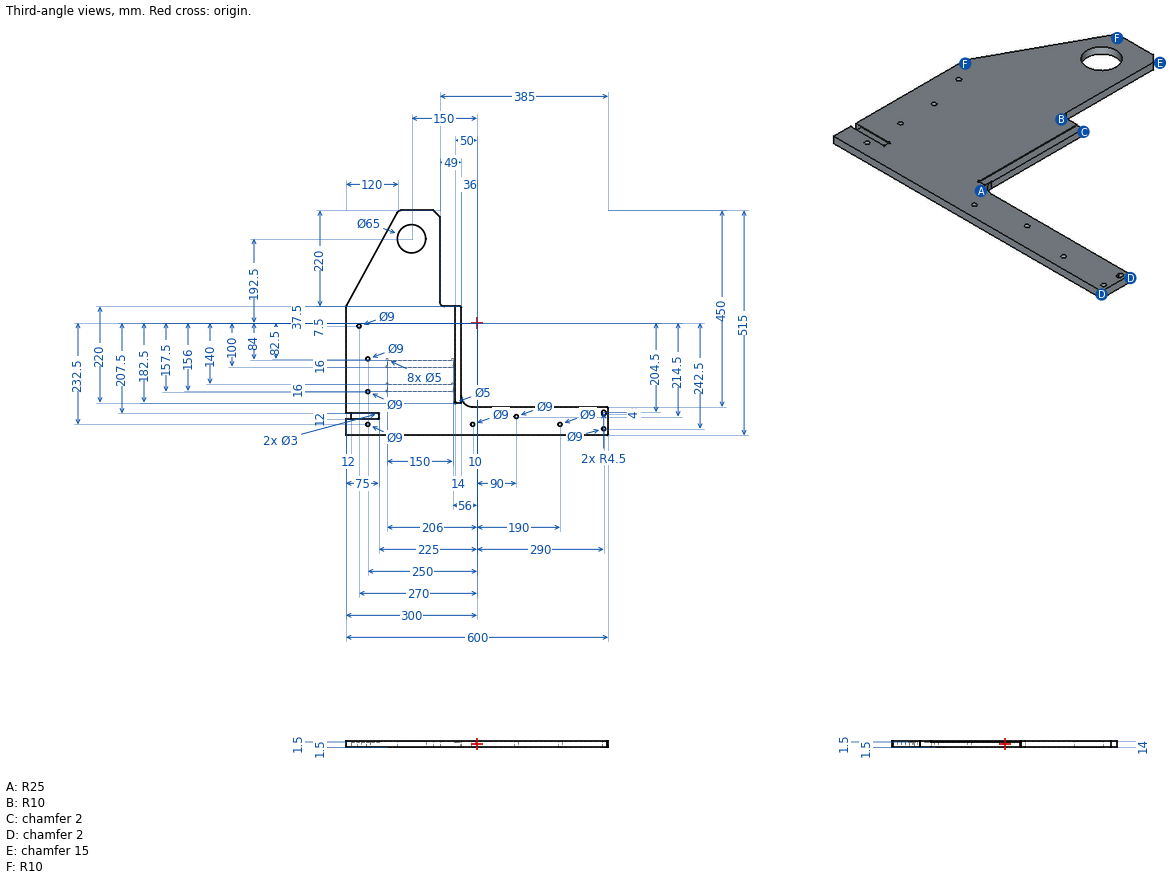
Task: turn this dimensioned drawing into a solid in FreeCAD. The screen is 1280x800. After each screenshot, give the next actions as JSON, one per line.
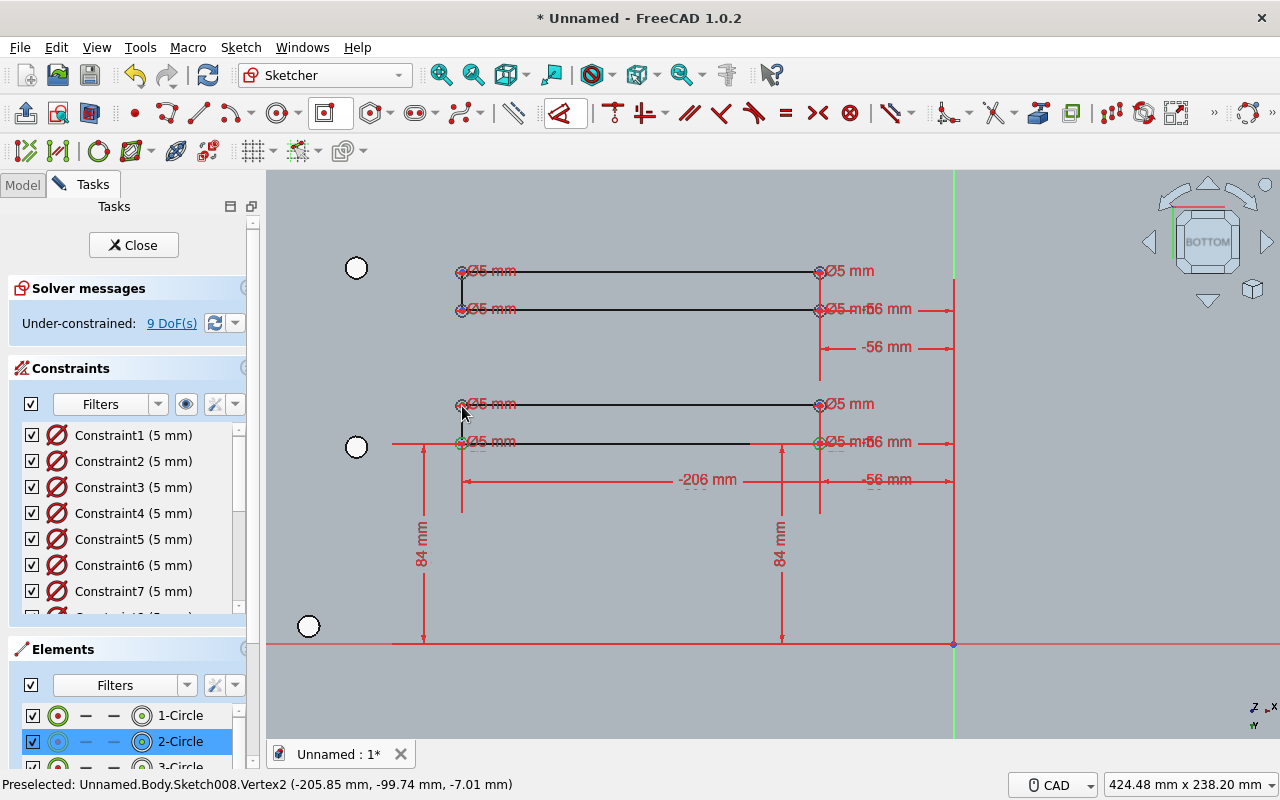
{"action": "left_click", "coordinate": [582, 114]}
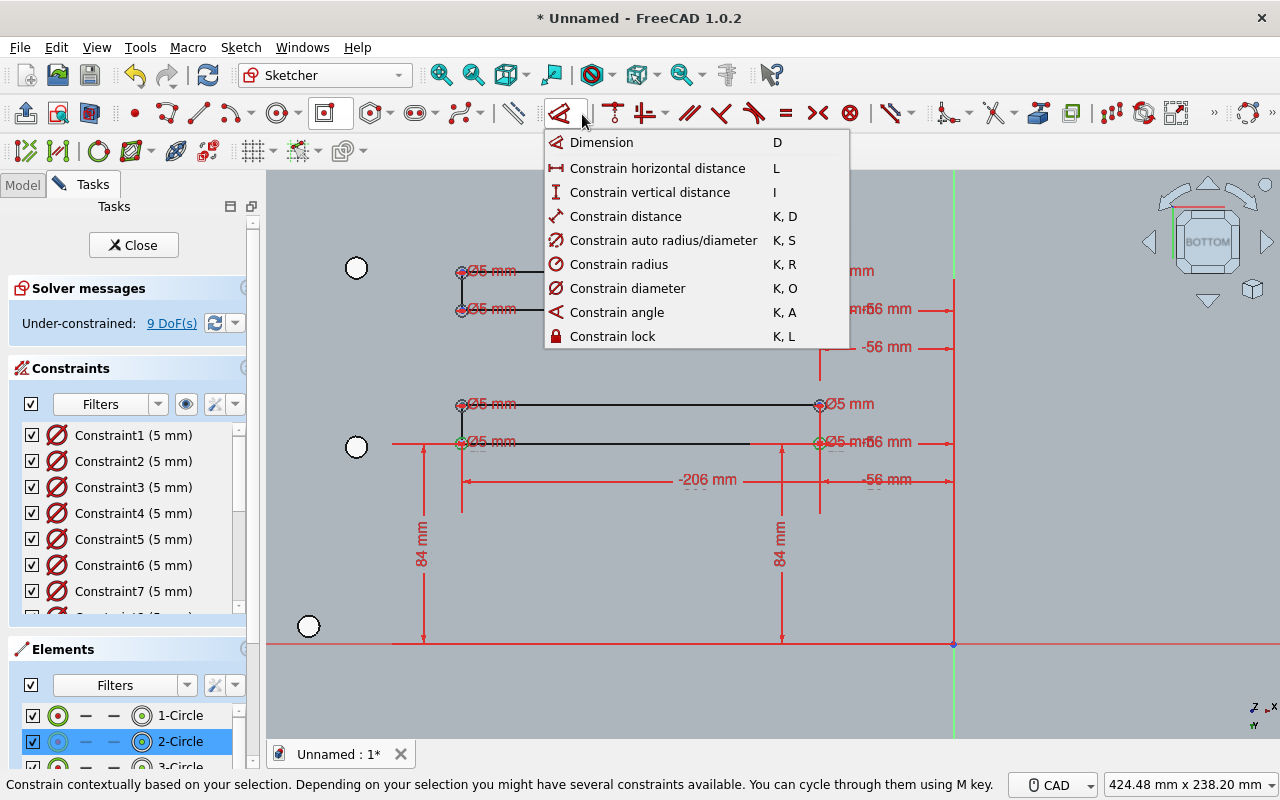
{"action": "left_click", "coordinate": [697, 168]}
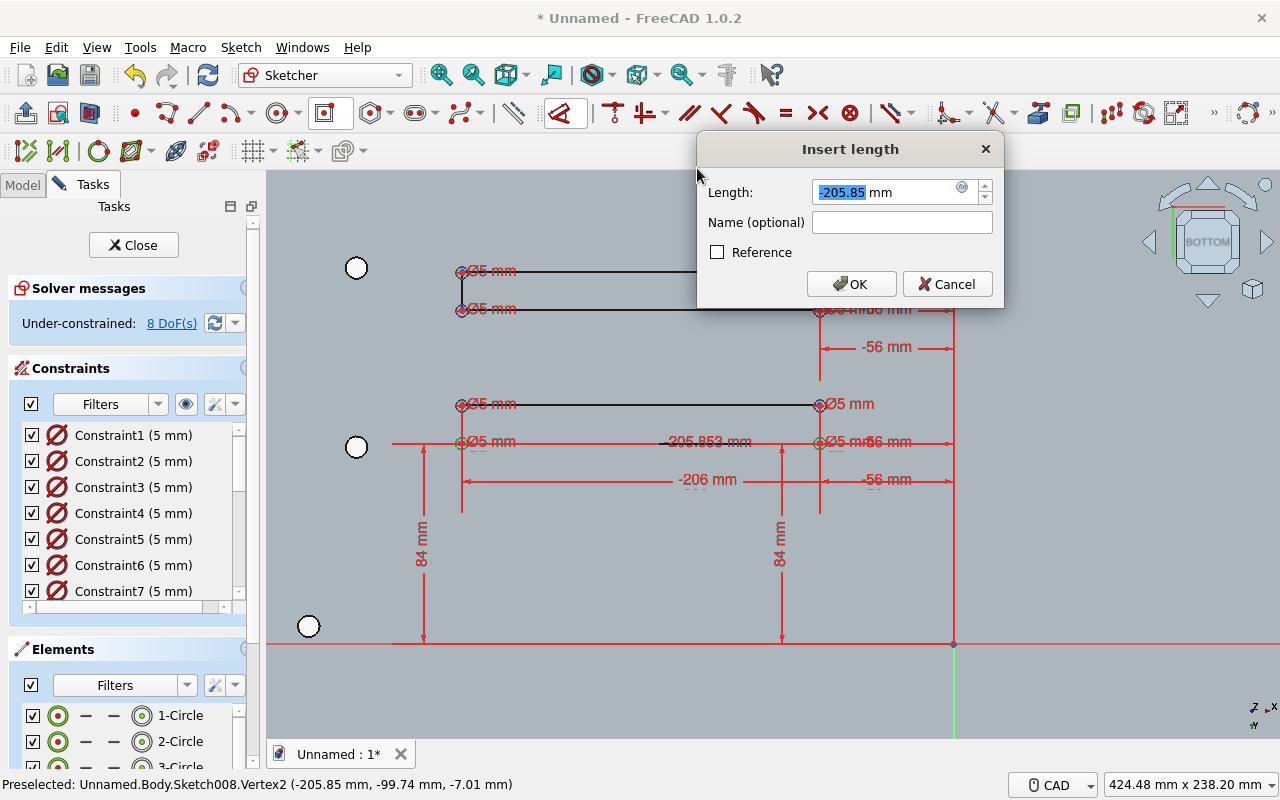
{"action": "type", "text": "-206"}
{"action": "key", "text": "Return"}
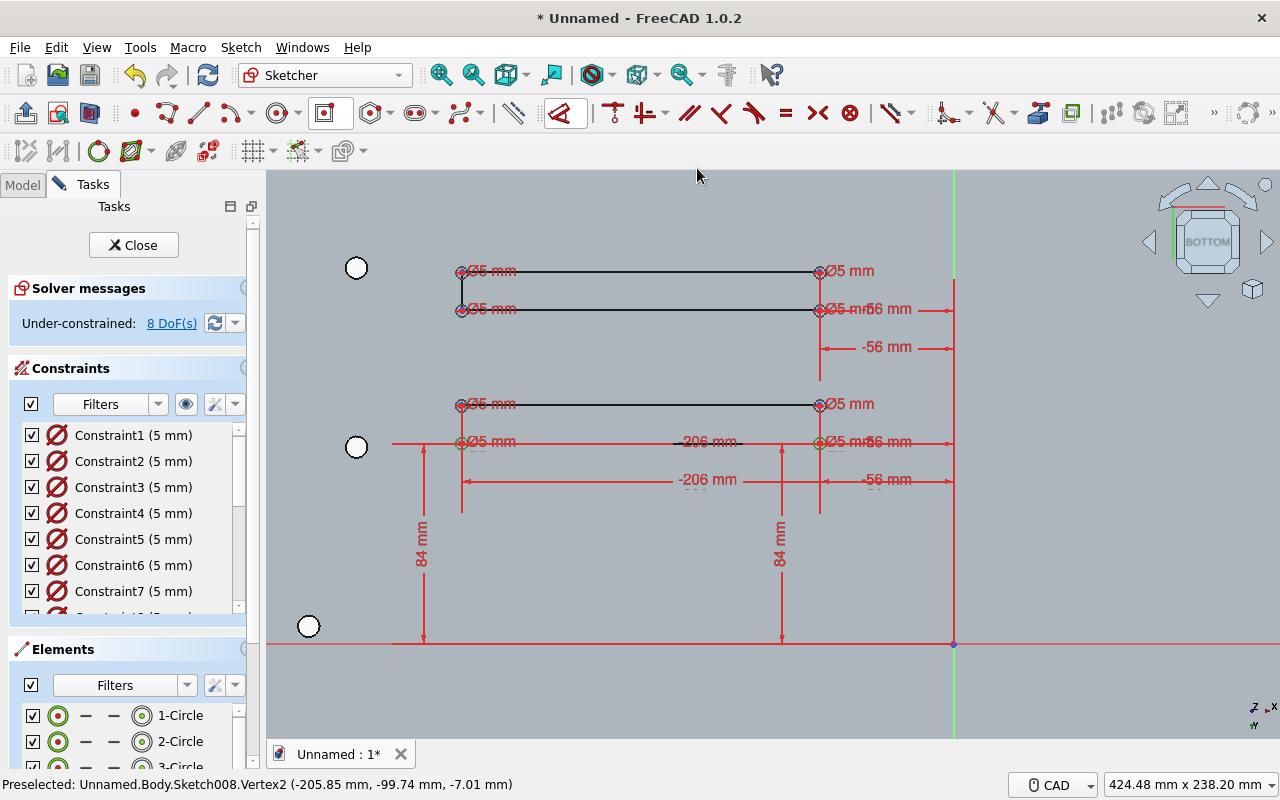
{"action": "left_click", "coordinate": [462, 406]}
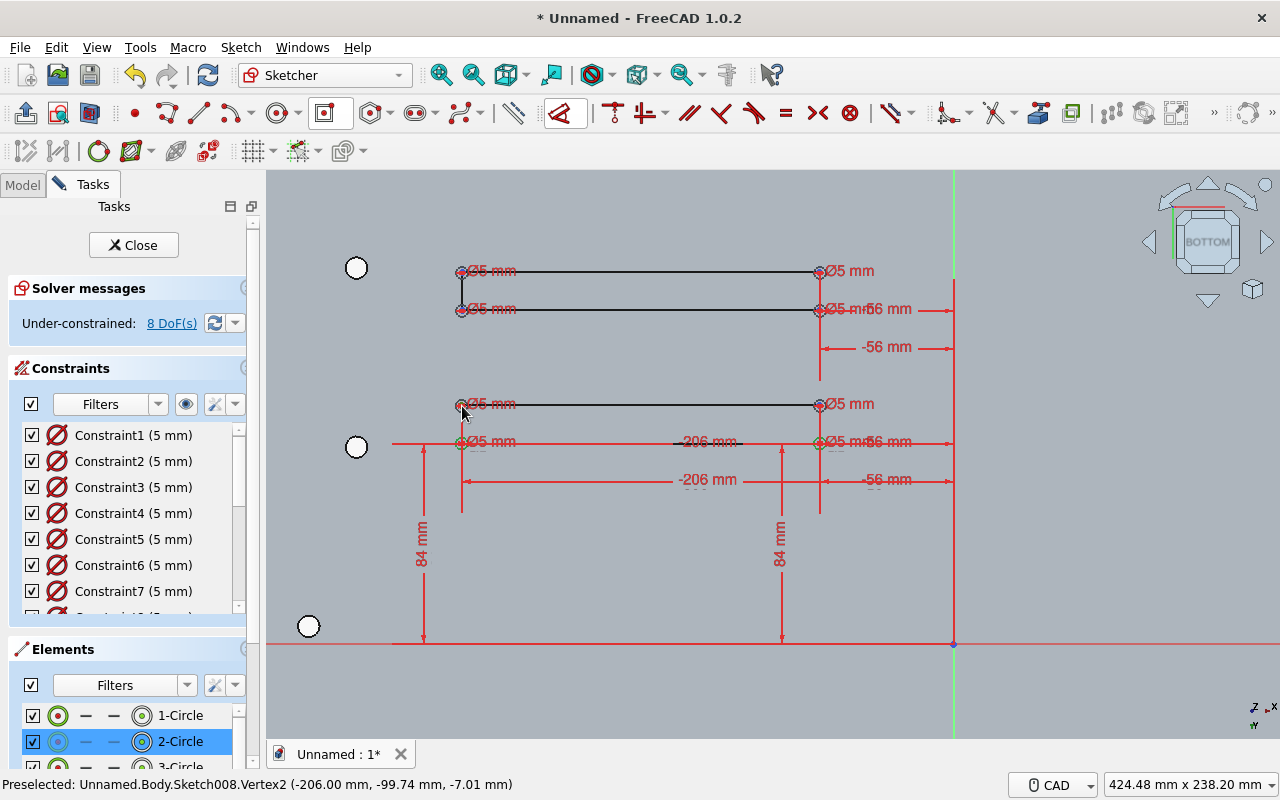
{"action": "left_click", "coordinate": [582, 114]}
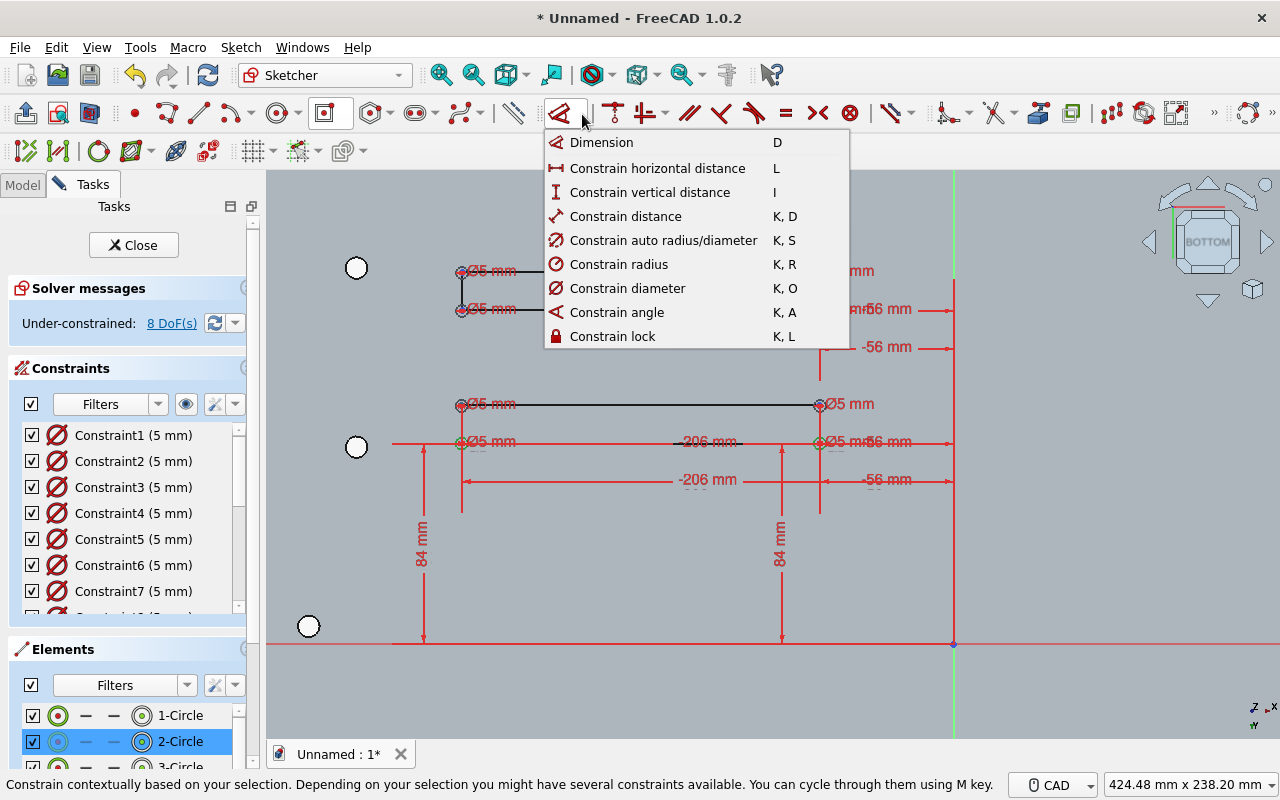
{"action": "left_click", "coordinate": [697, 192]}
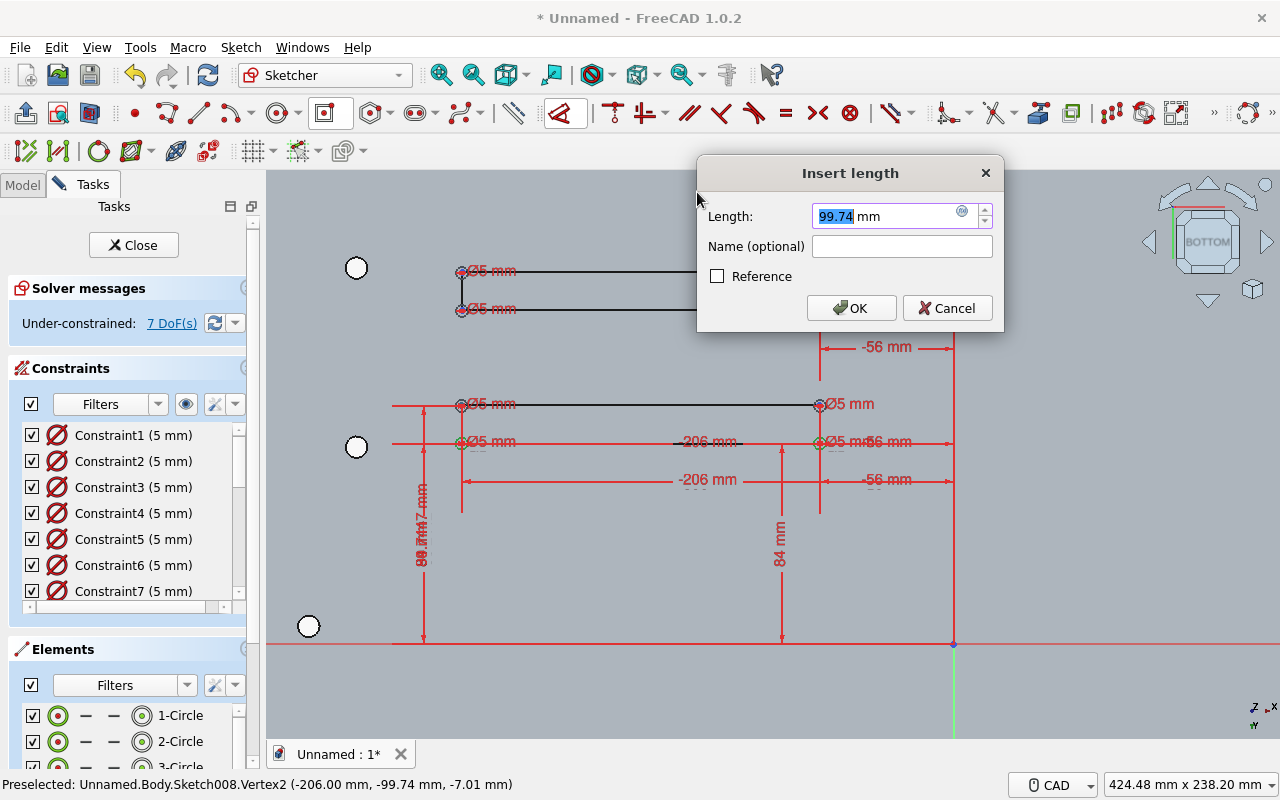
{"action": "type", "text": "100"}
{"action": "key", "text": "Return"}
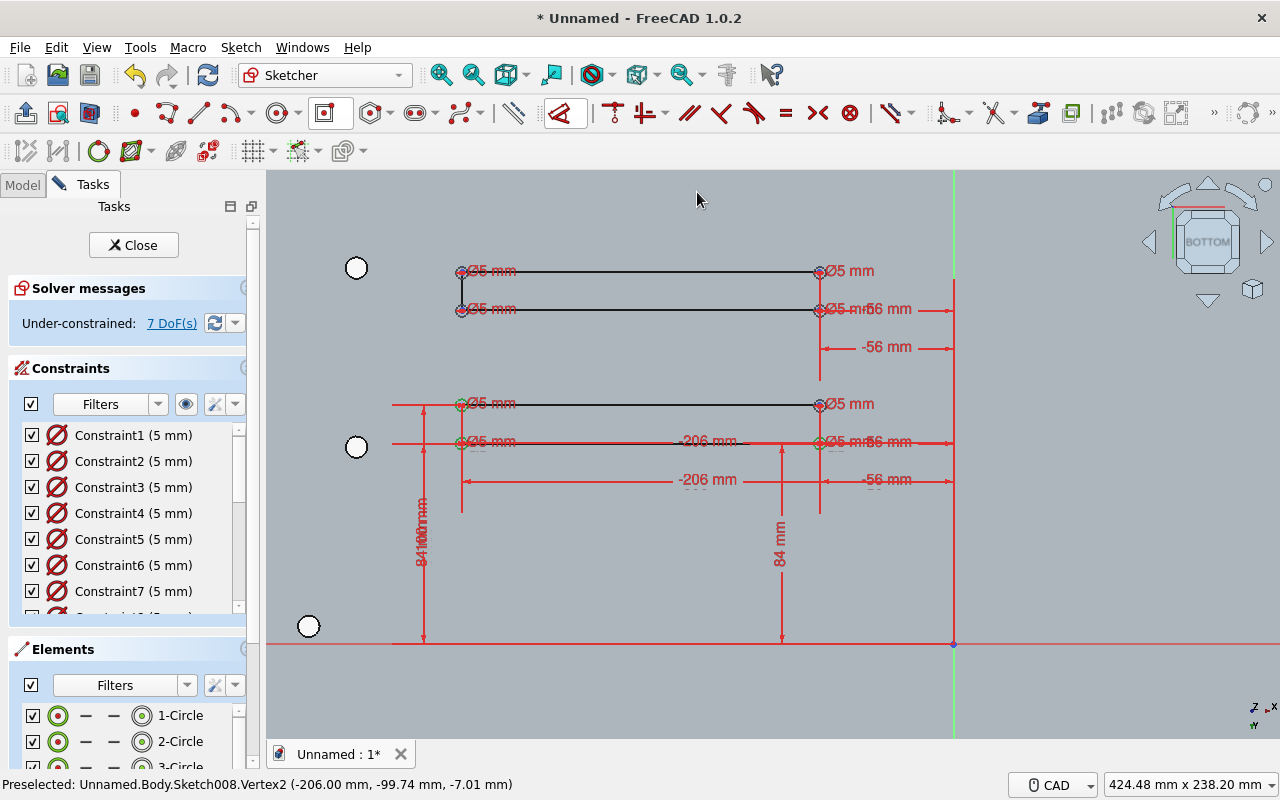
{"action": "left_click", "coordinate": [462, 311]}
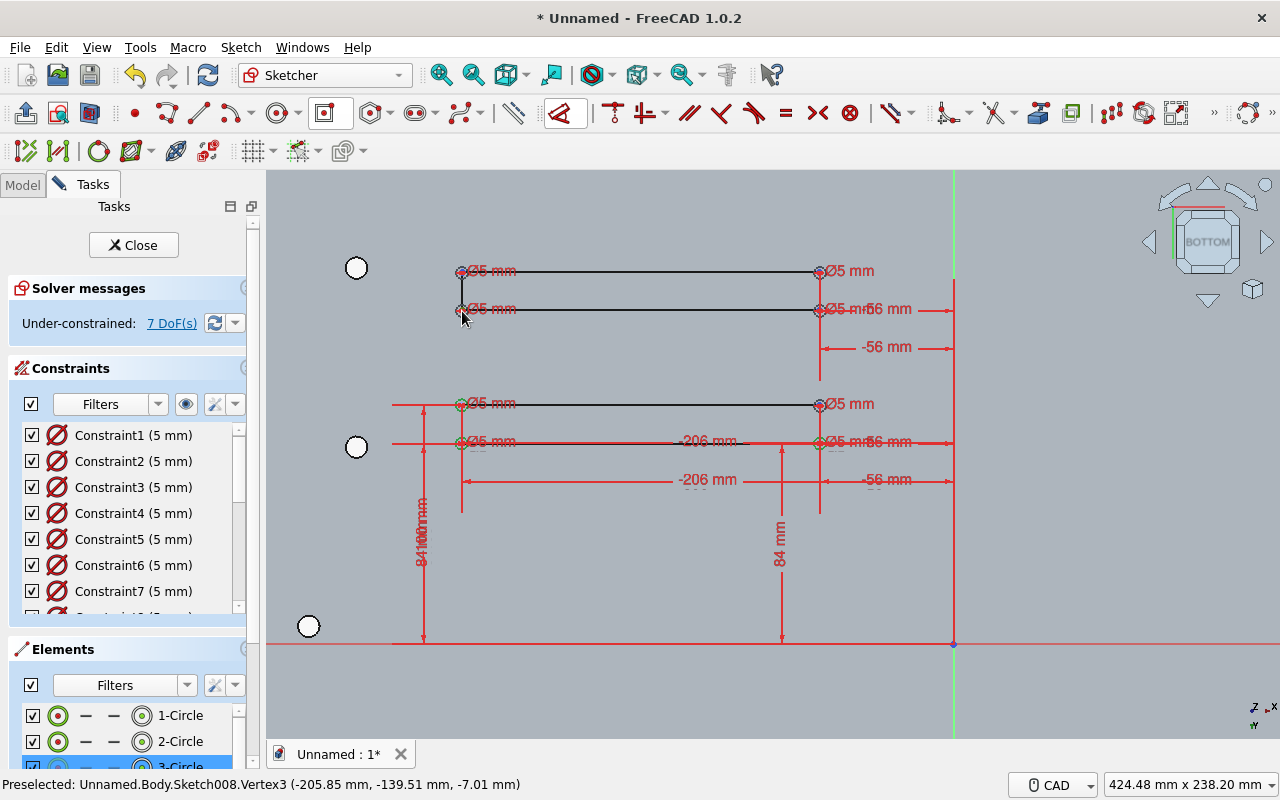
{"action": "left_click", "coordinate": [582, 114]}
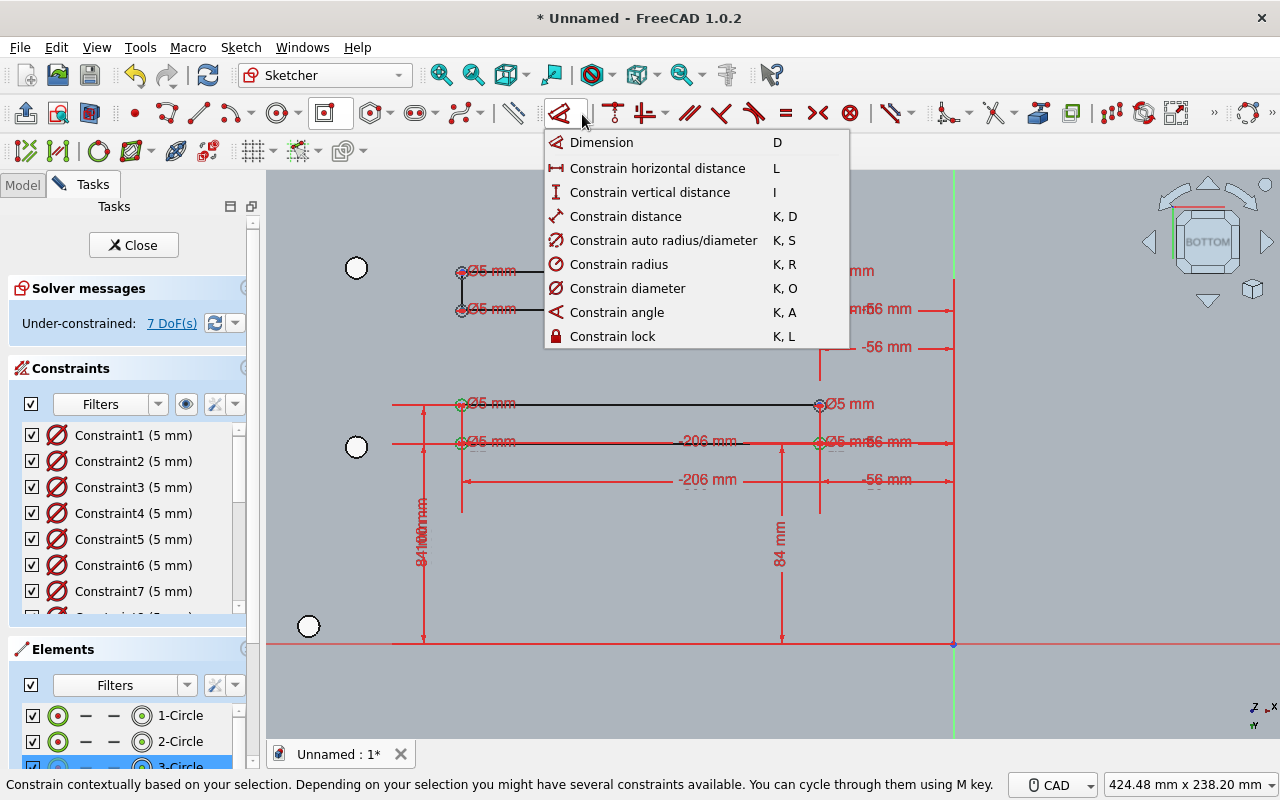
{"action": "left_click", "coordinate": [697, 168]}